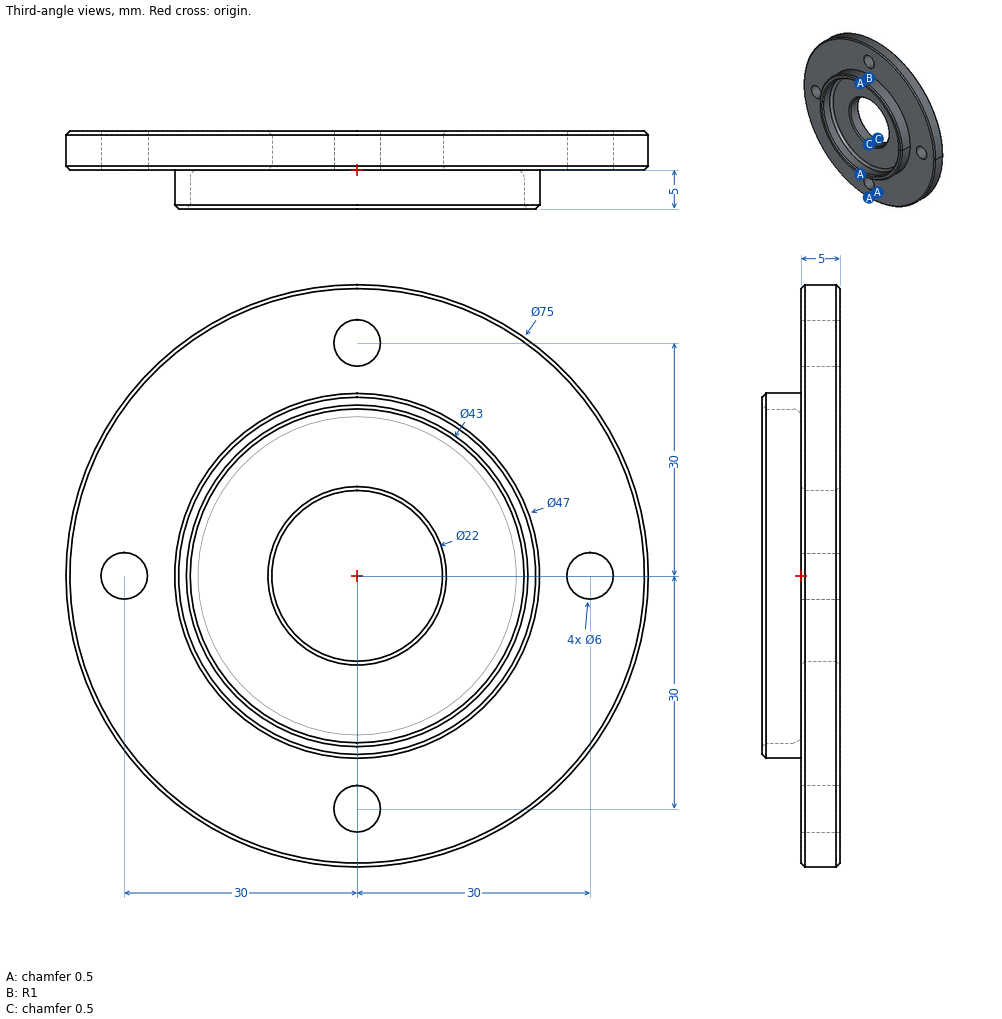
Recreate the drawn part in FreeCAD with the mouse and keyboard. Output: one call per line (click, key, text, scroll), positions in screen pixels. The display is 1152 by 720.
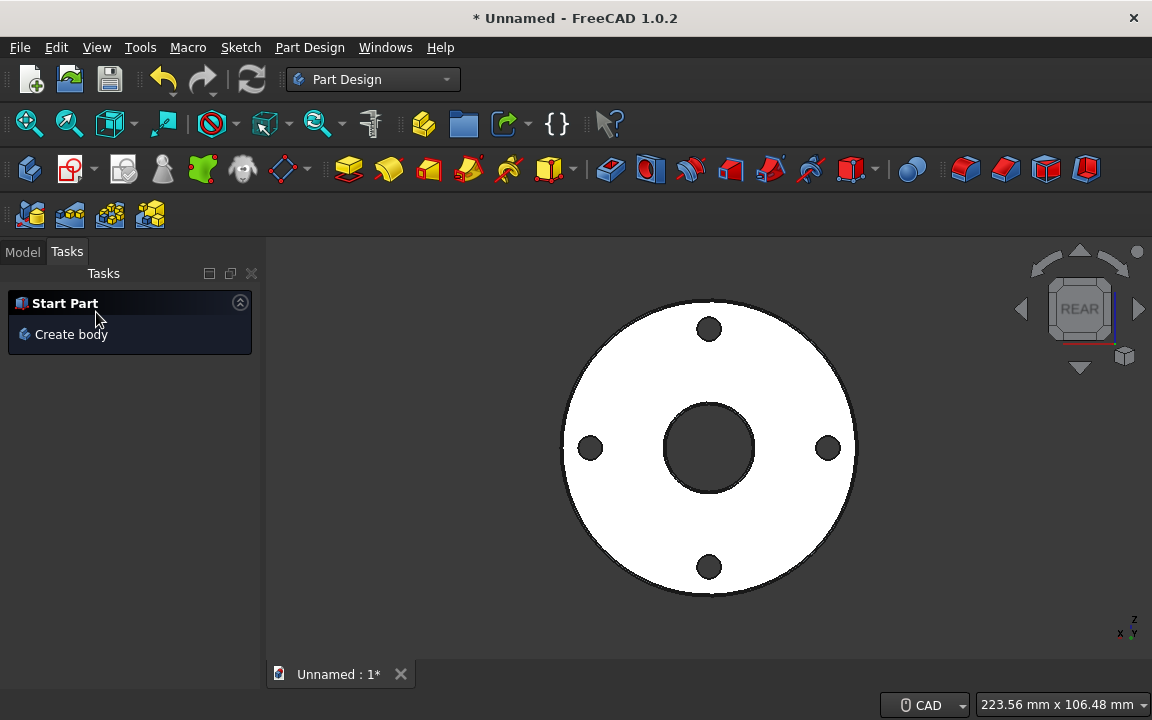
key(0)